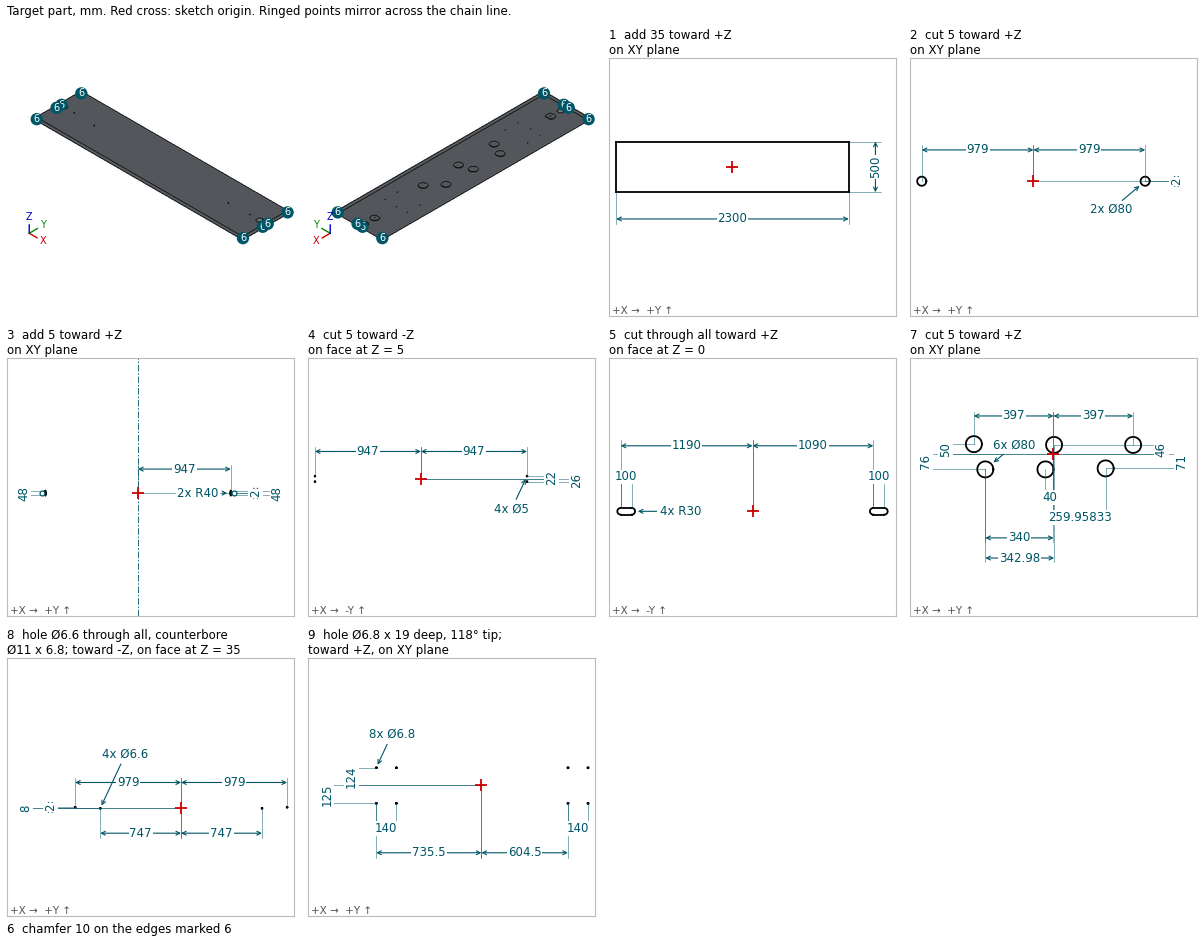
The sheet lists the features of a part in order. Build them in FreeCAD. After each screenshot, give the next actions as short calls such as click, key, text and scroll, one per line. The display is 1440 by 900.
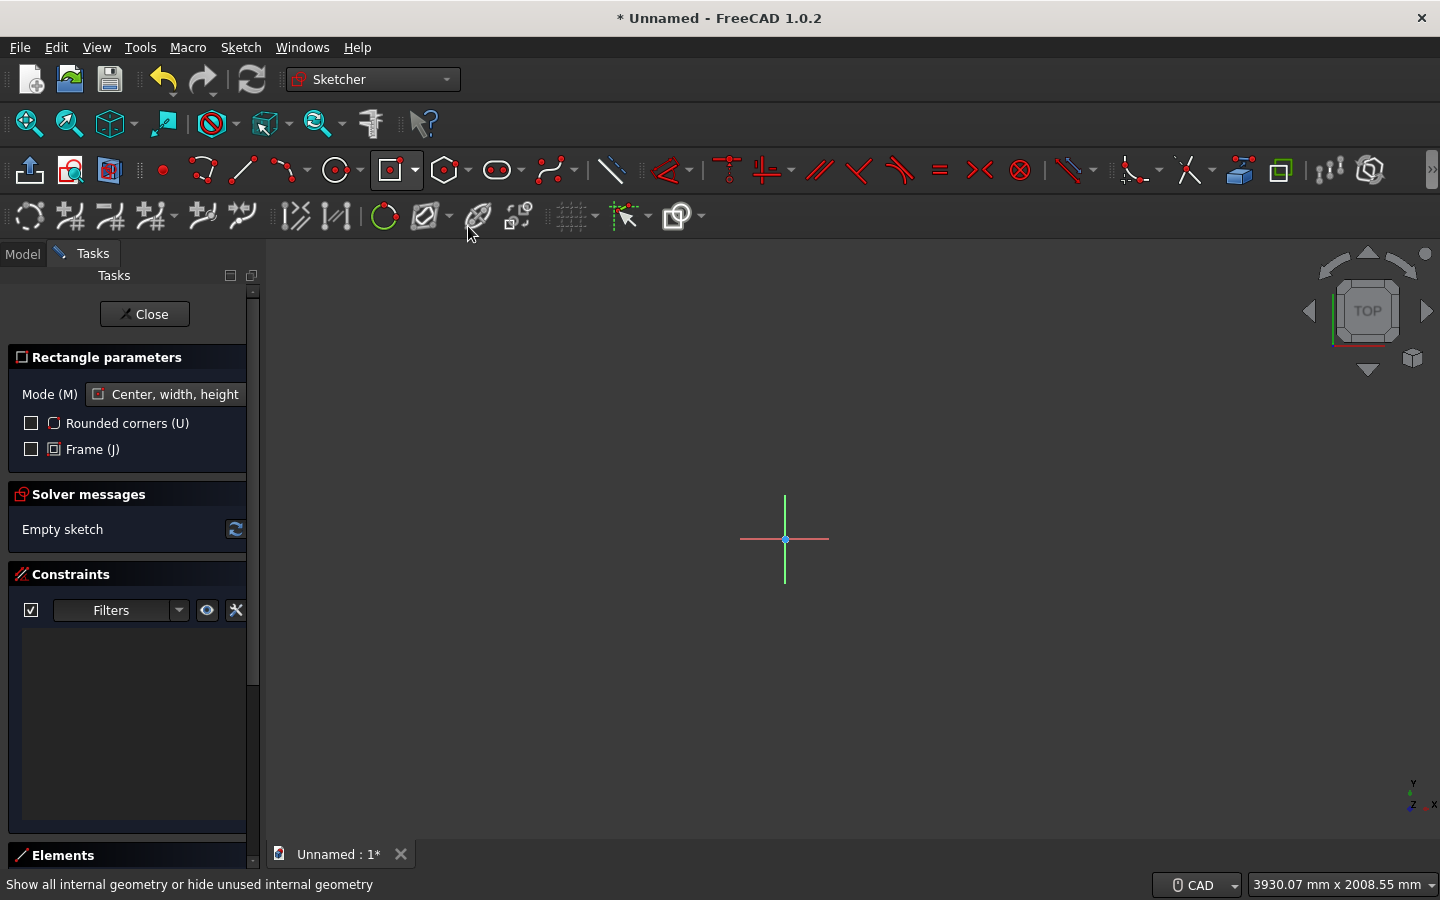
click(785, 539)
click(1129, 465)
key(Escape)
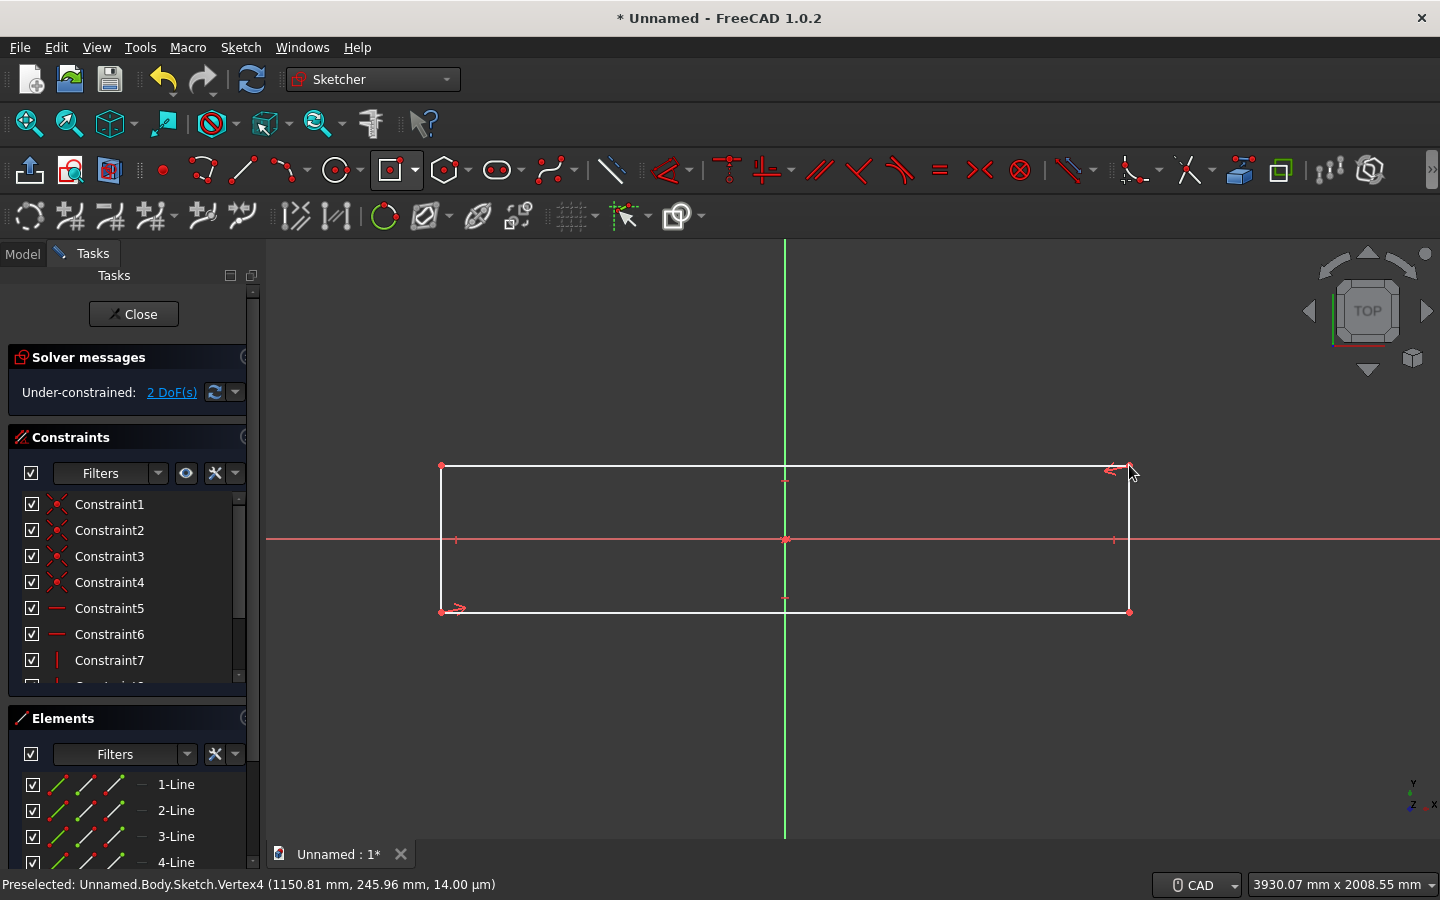
click(666, 170)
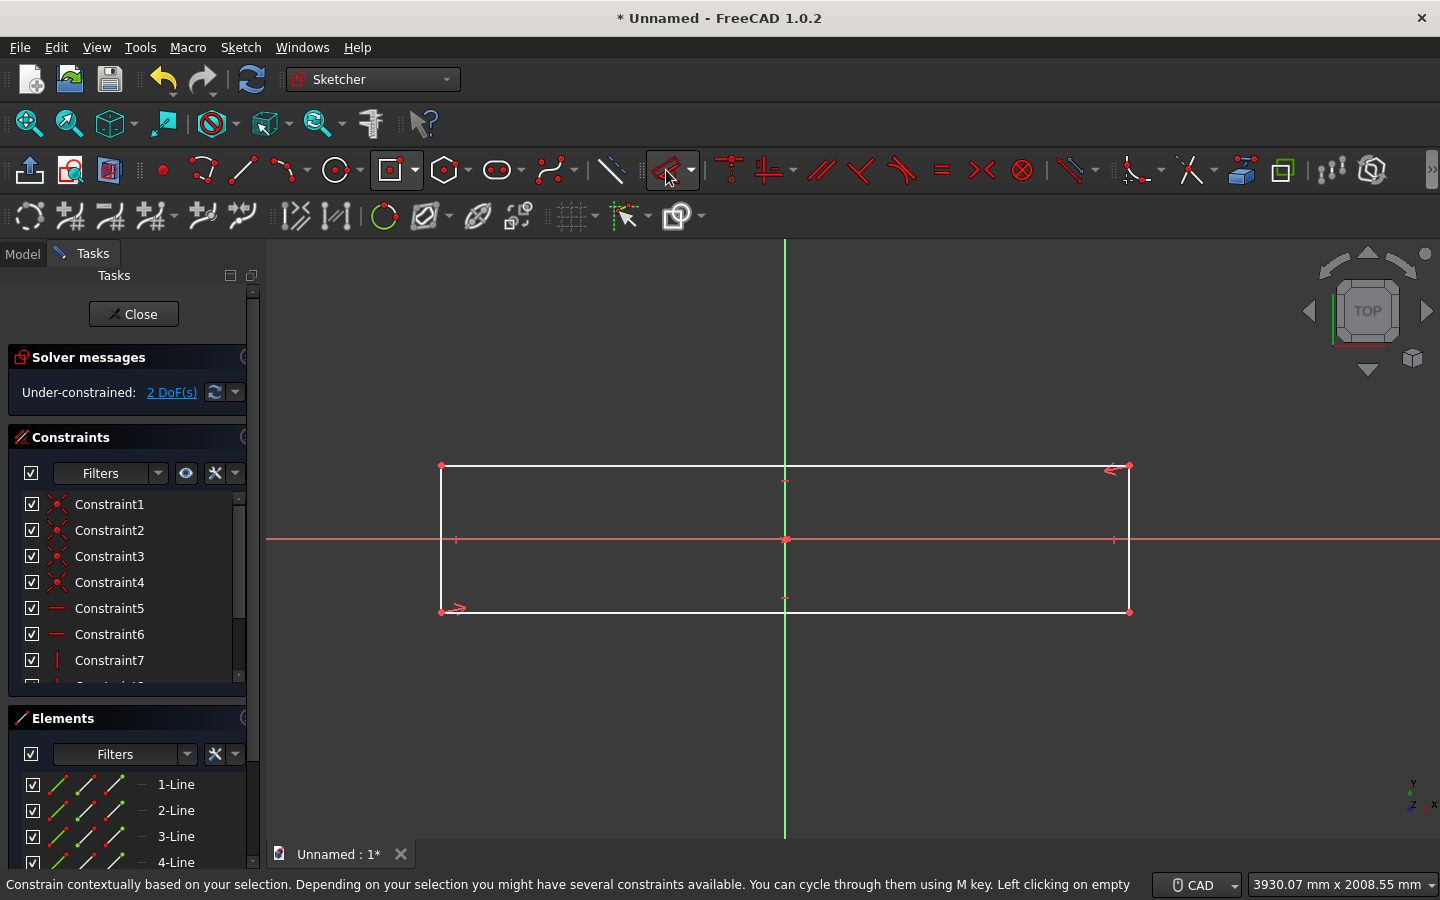
click(1129, 569)
click(1163, 506)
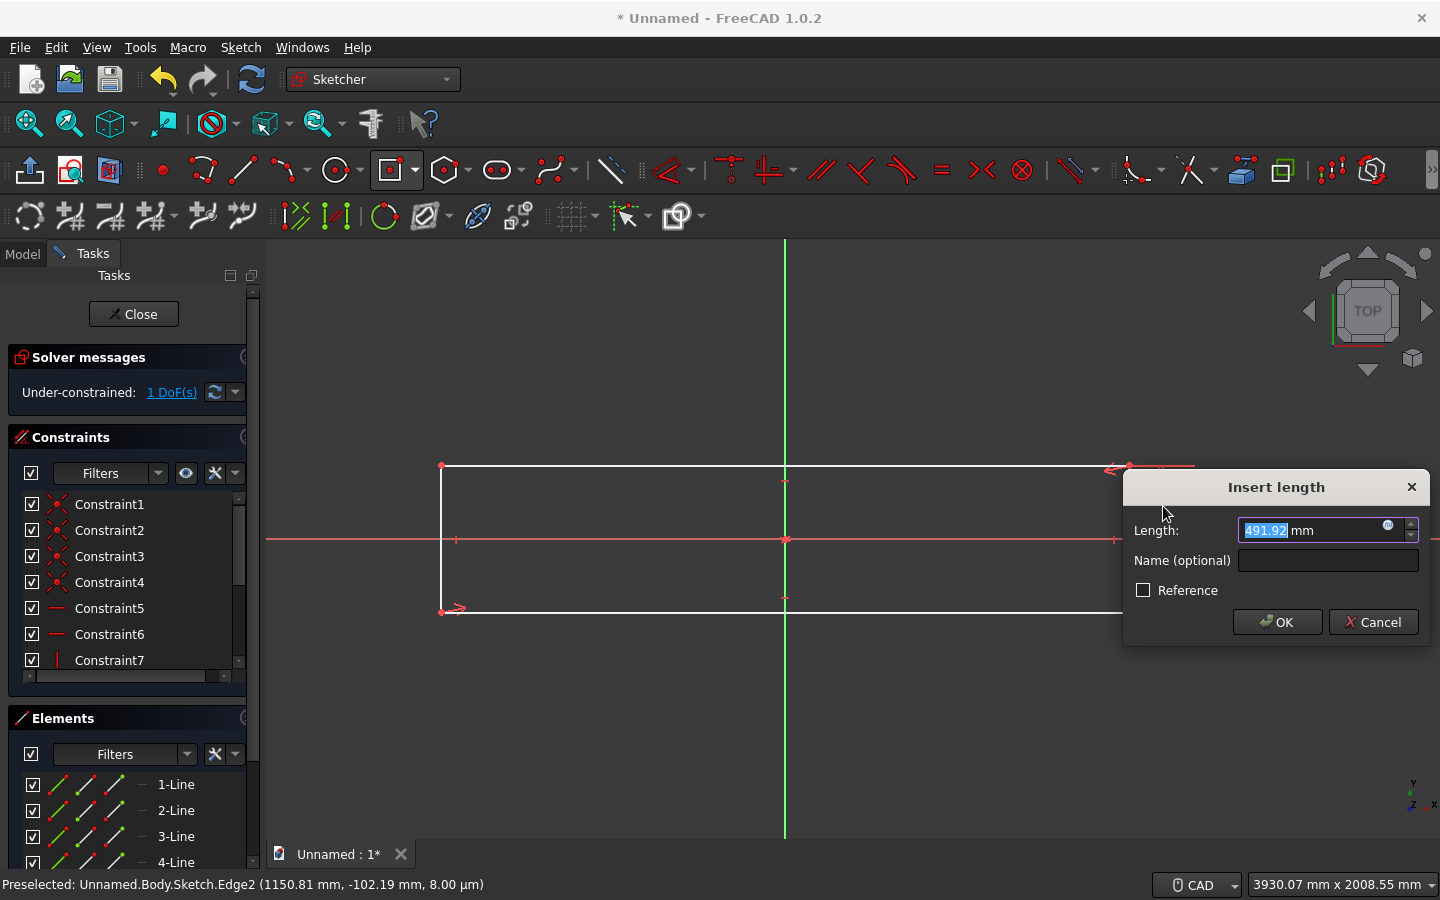
text(500)
key(Return)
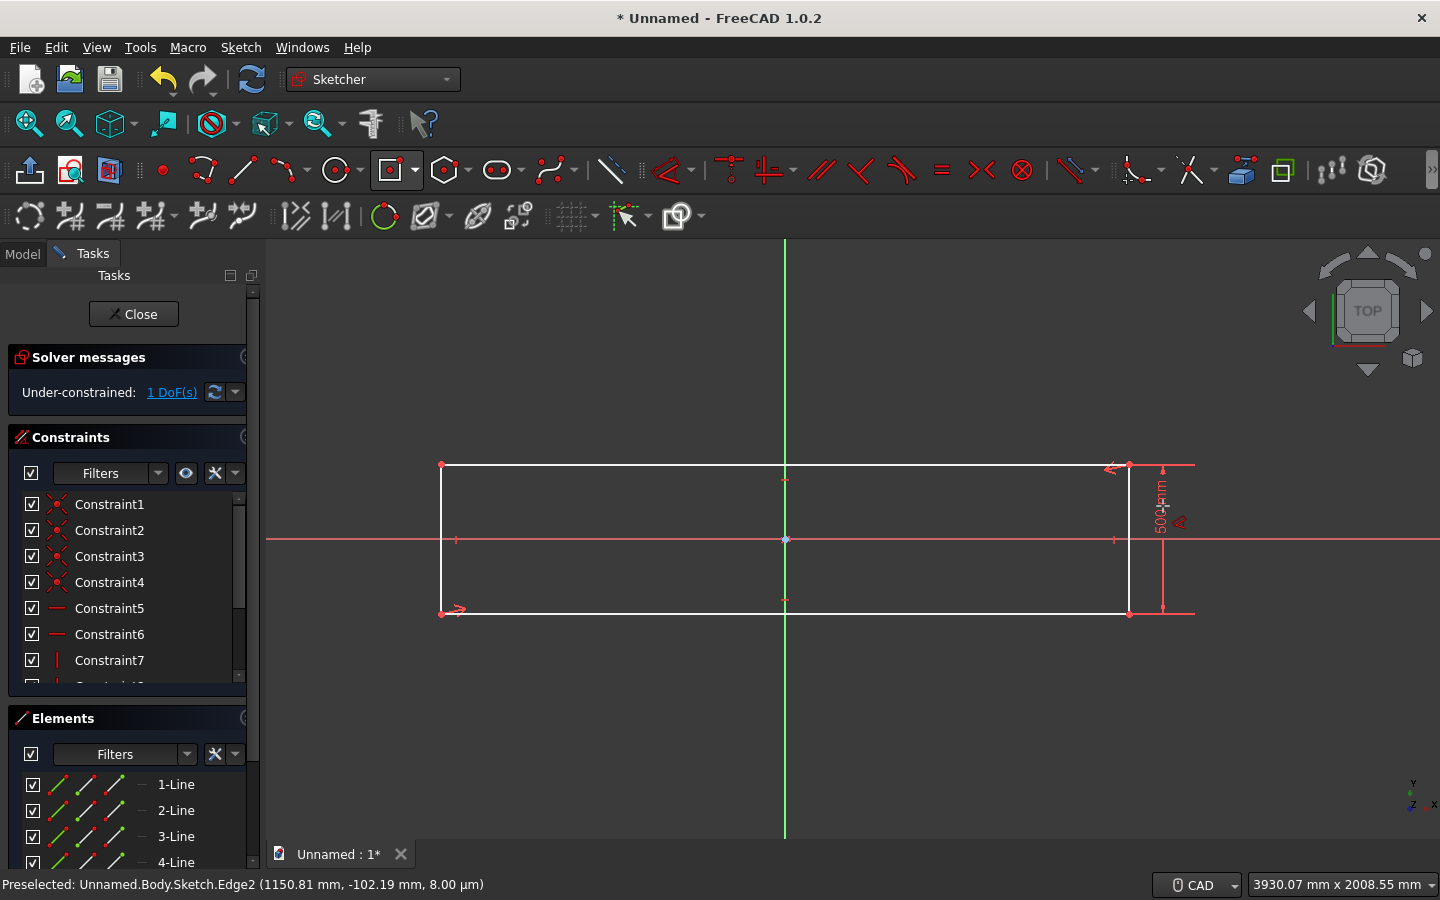
click(648, 614)
click(627, 648)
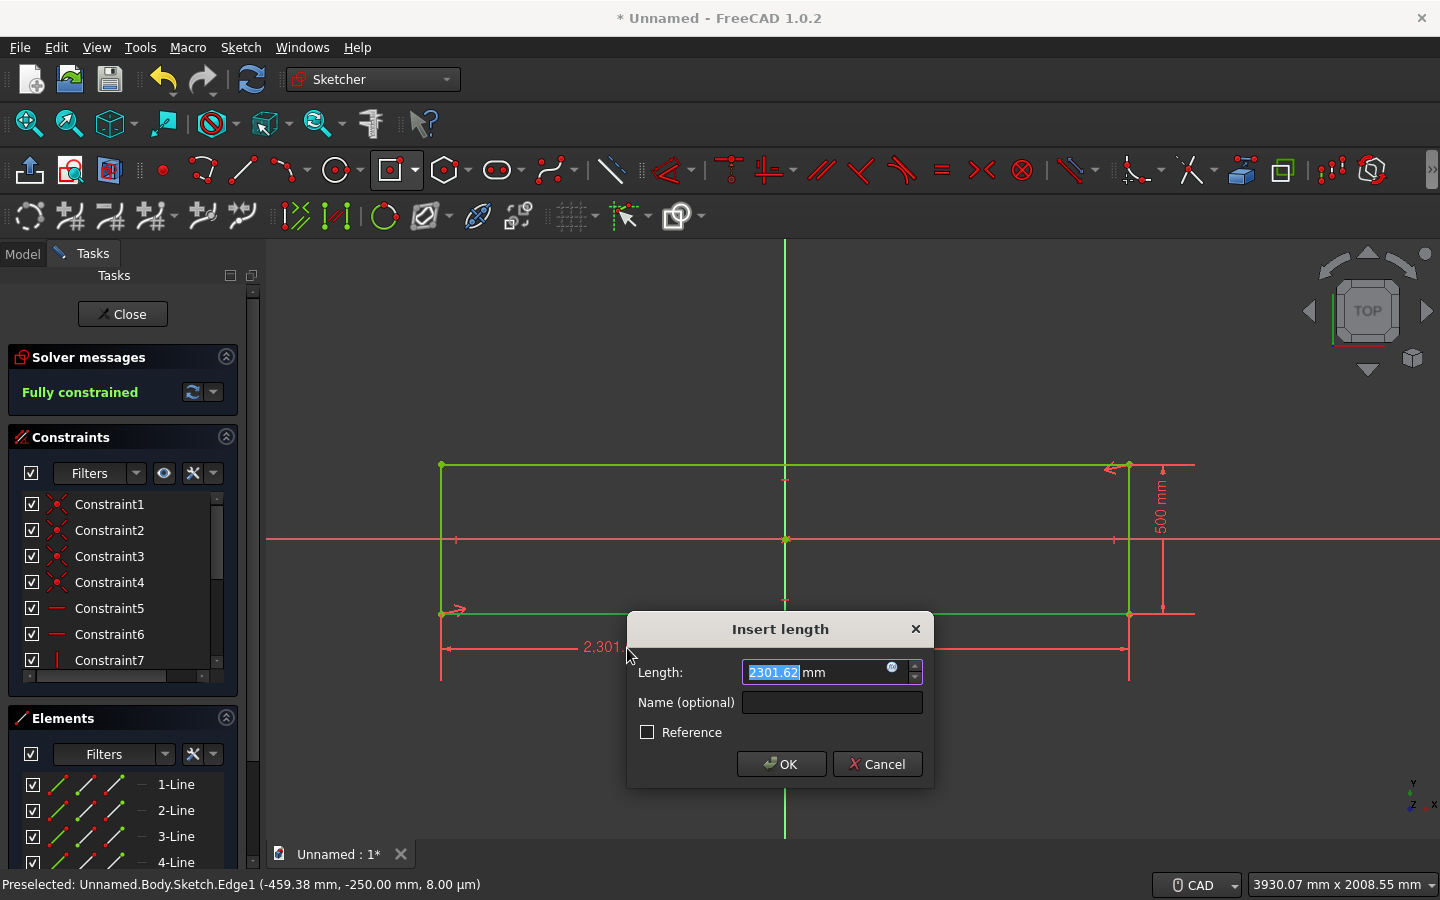
text(2300)
key(Return)
key(Escape)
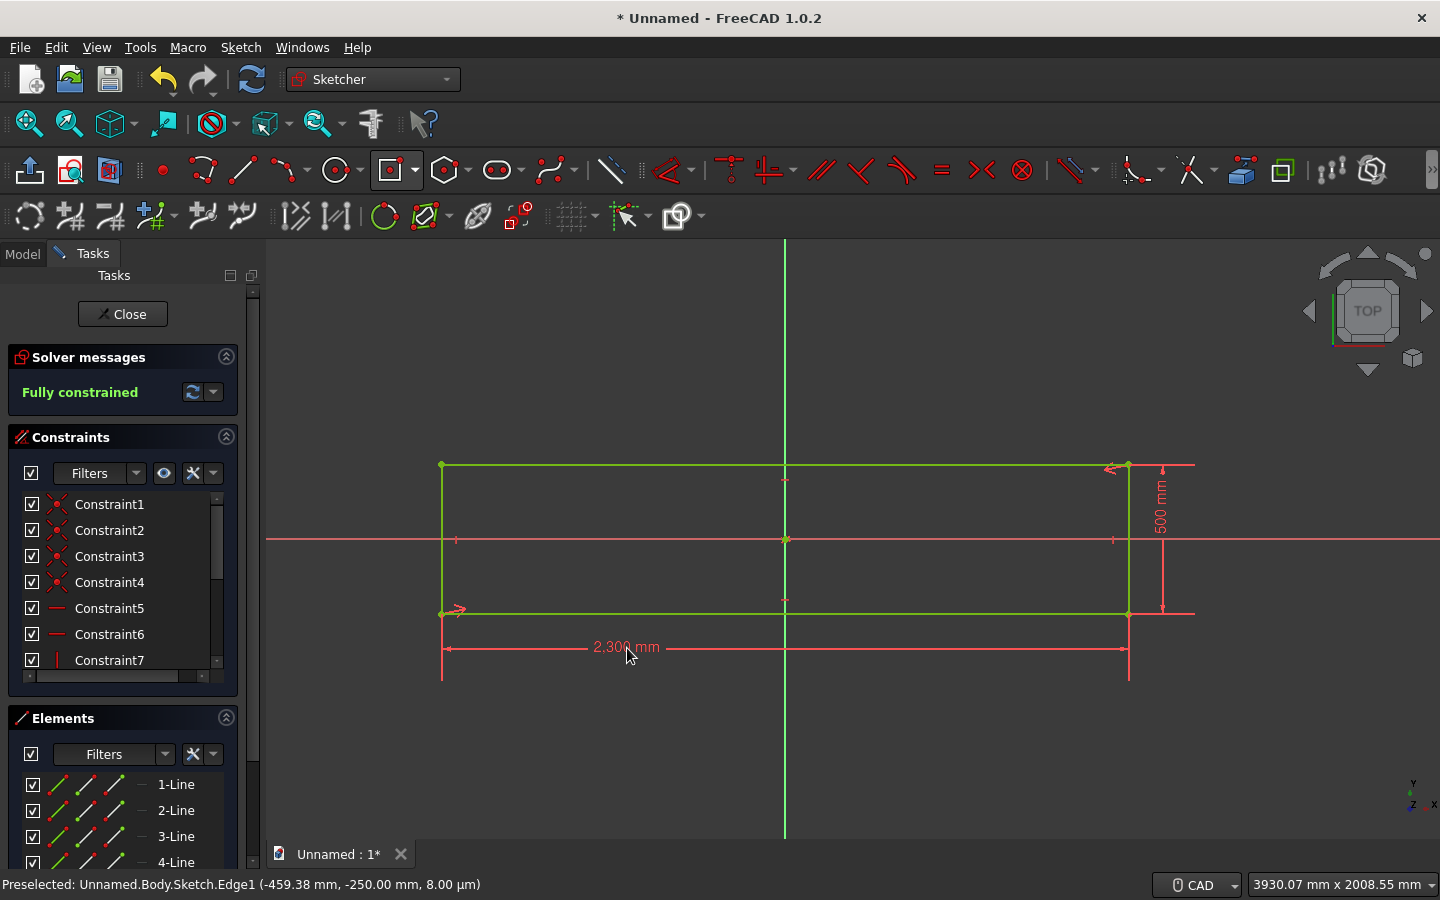
click(123, 314)